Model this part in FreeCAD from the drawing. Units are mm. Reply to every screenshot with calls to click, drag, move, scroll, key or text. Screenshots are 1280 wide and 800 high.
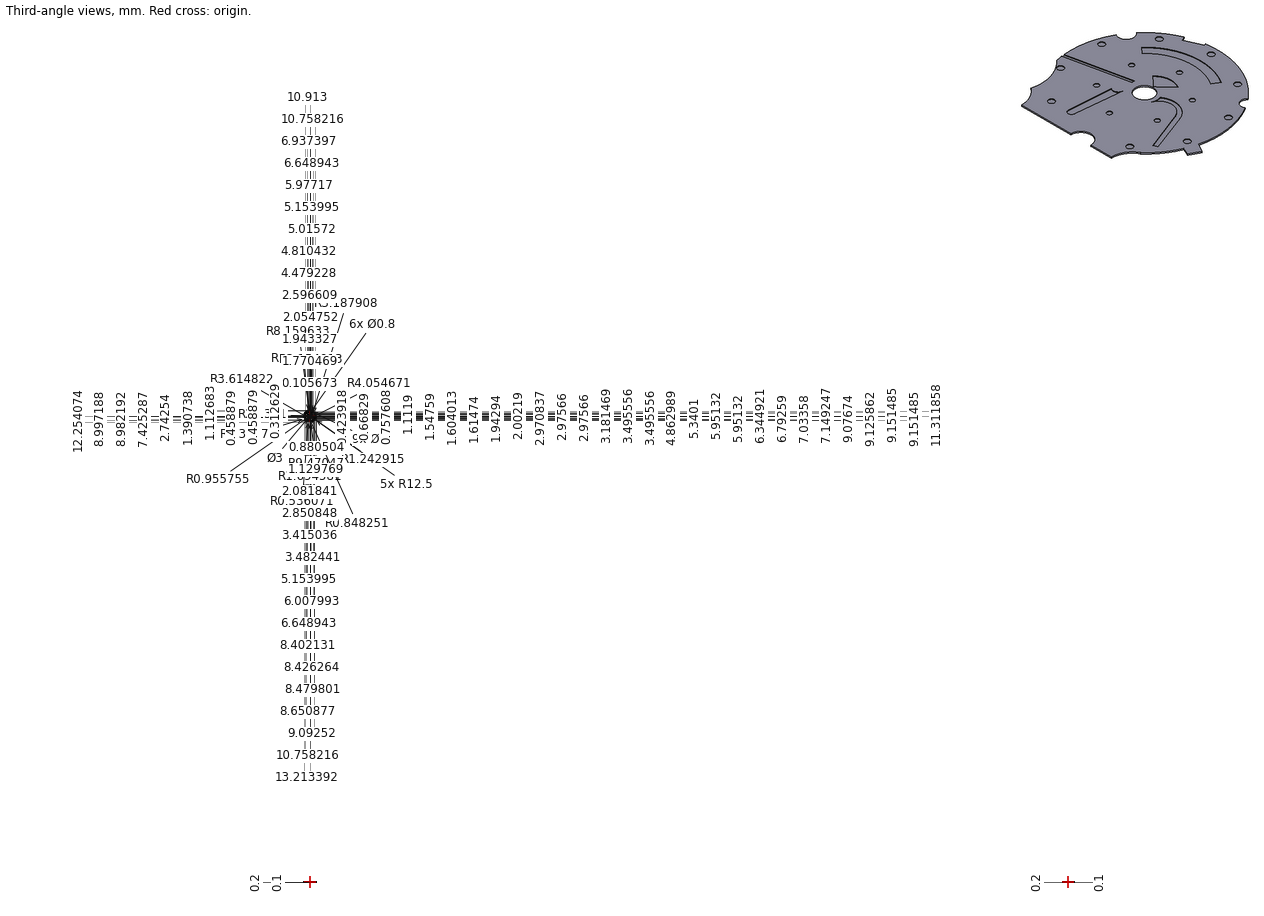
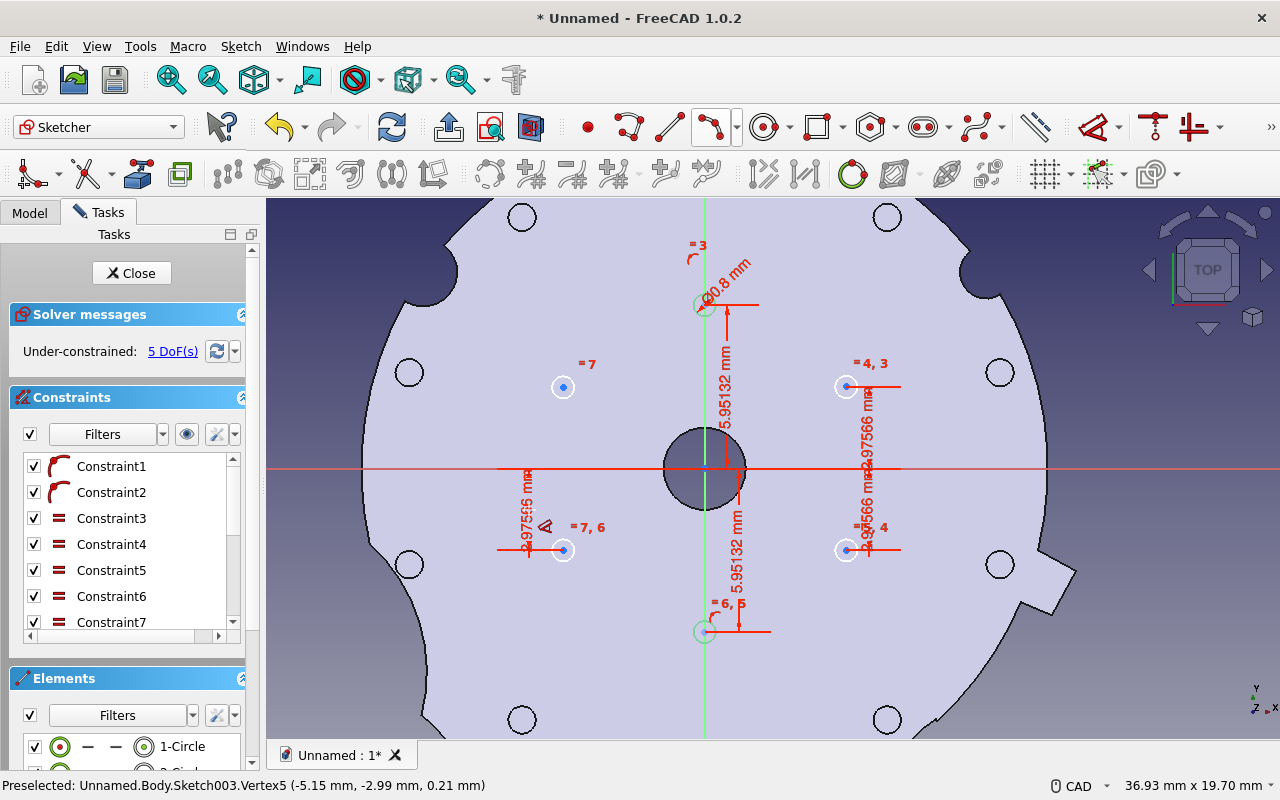
click(563, 387)
click(529, 428)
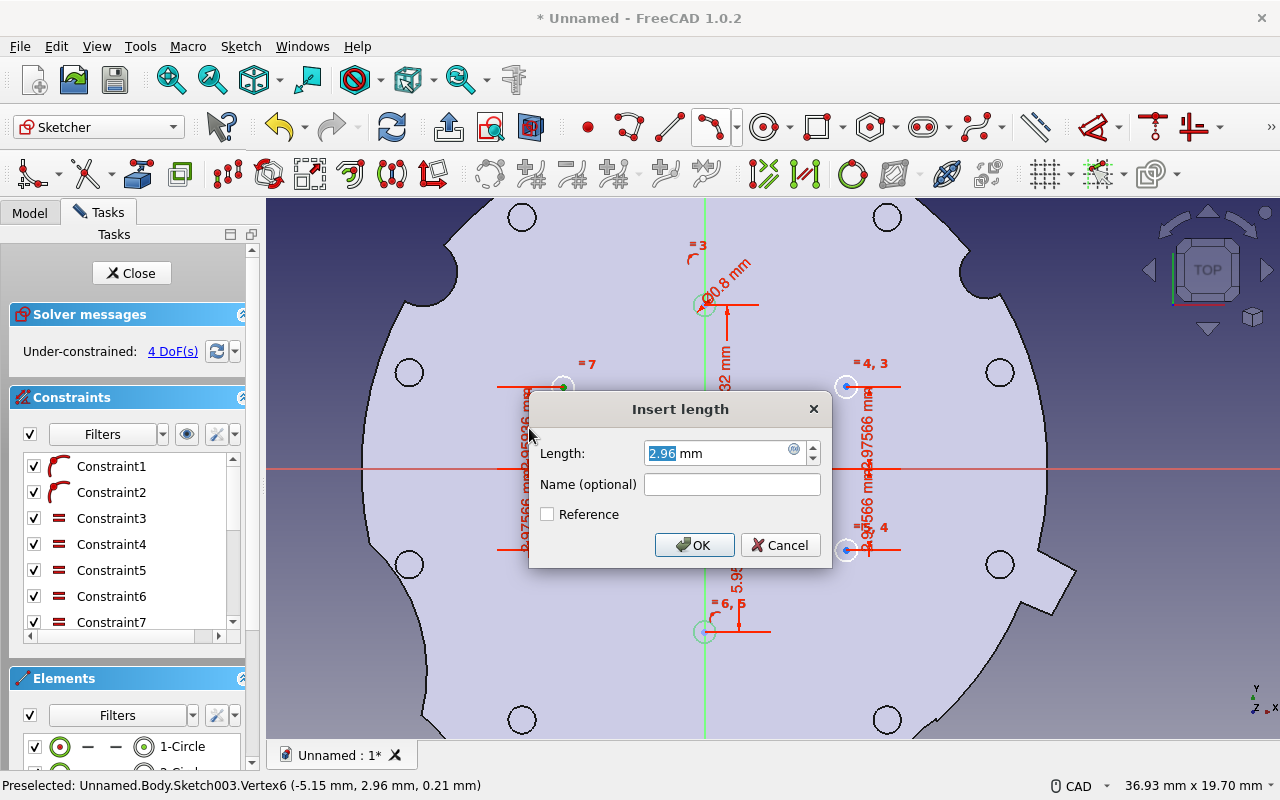
text(2.97566)
key(Return)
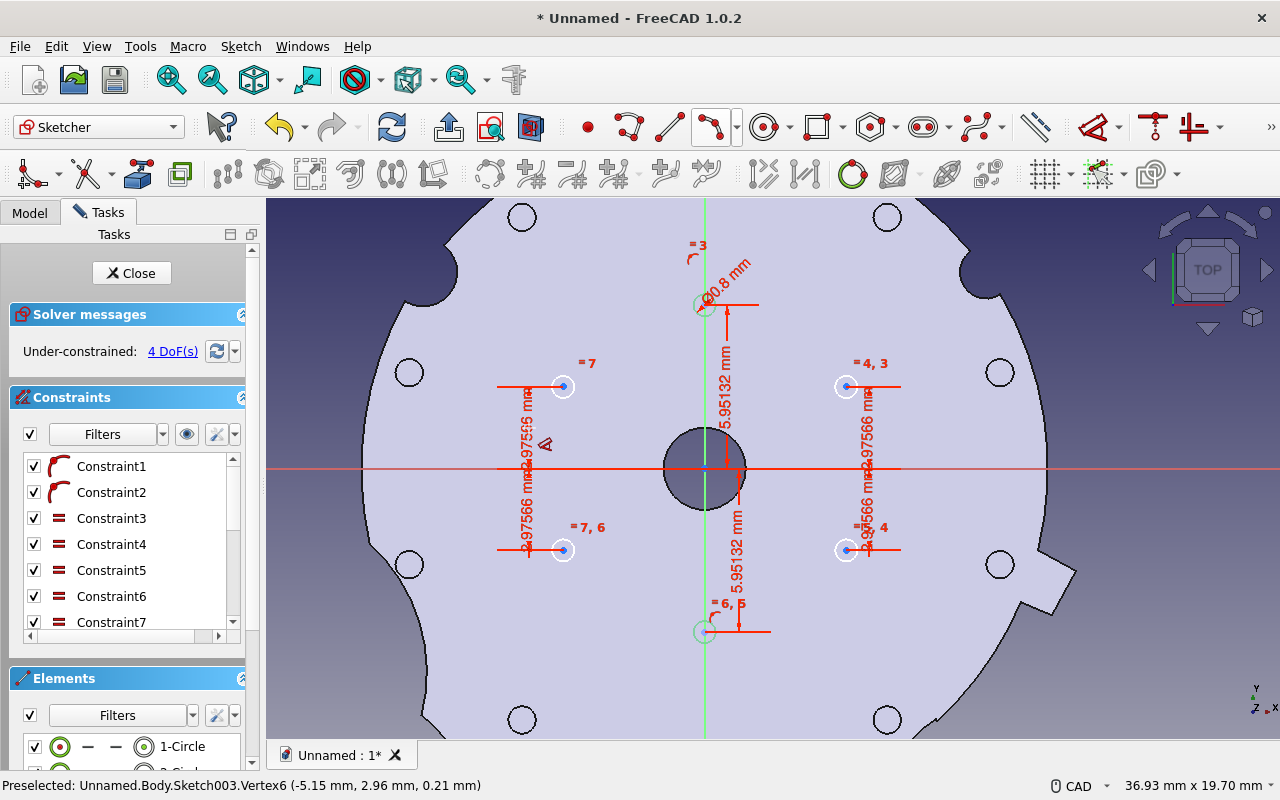
click(846, 387)
click(775, 353)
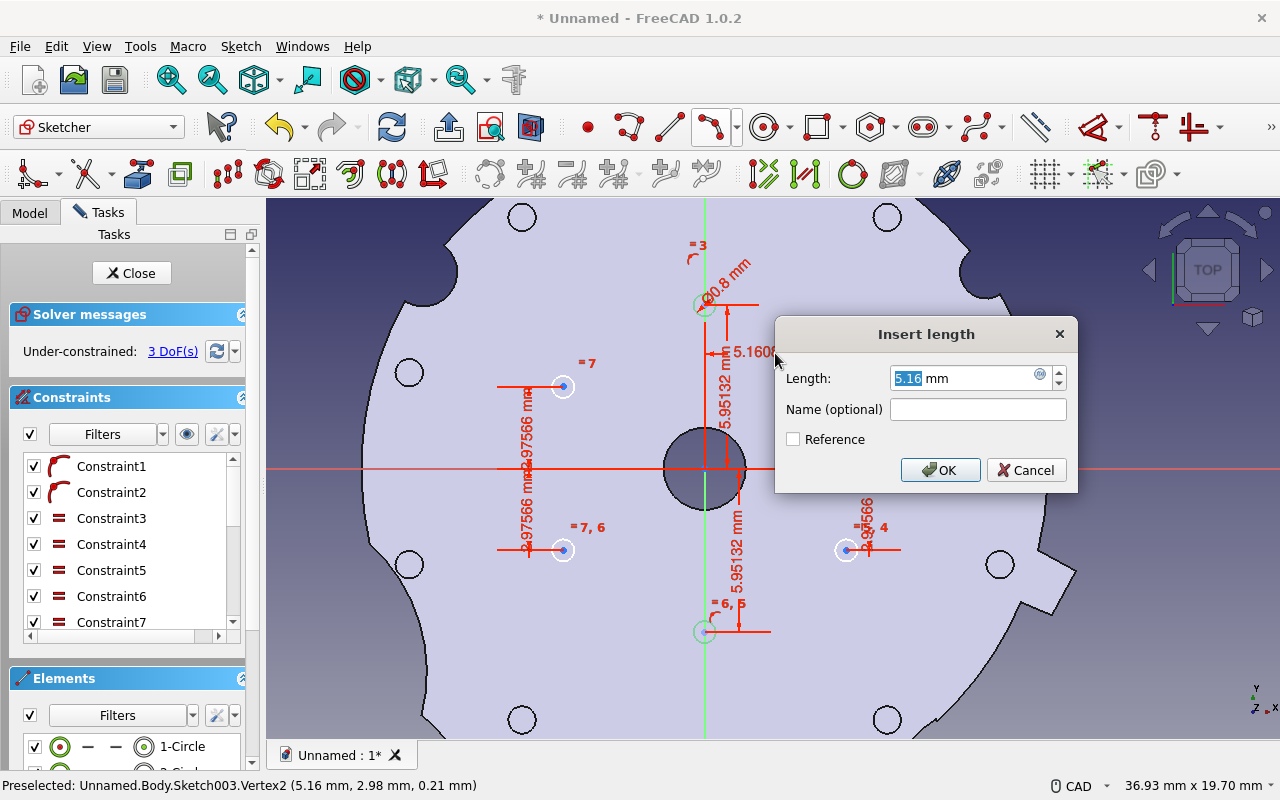
text(5.153995)
key(Return)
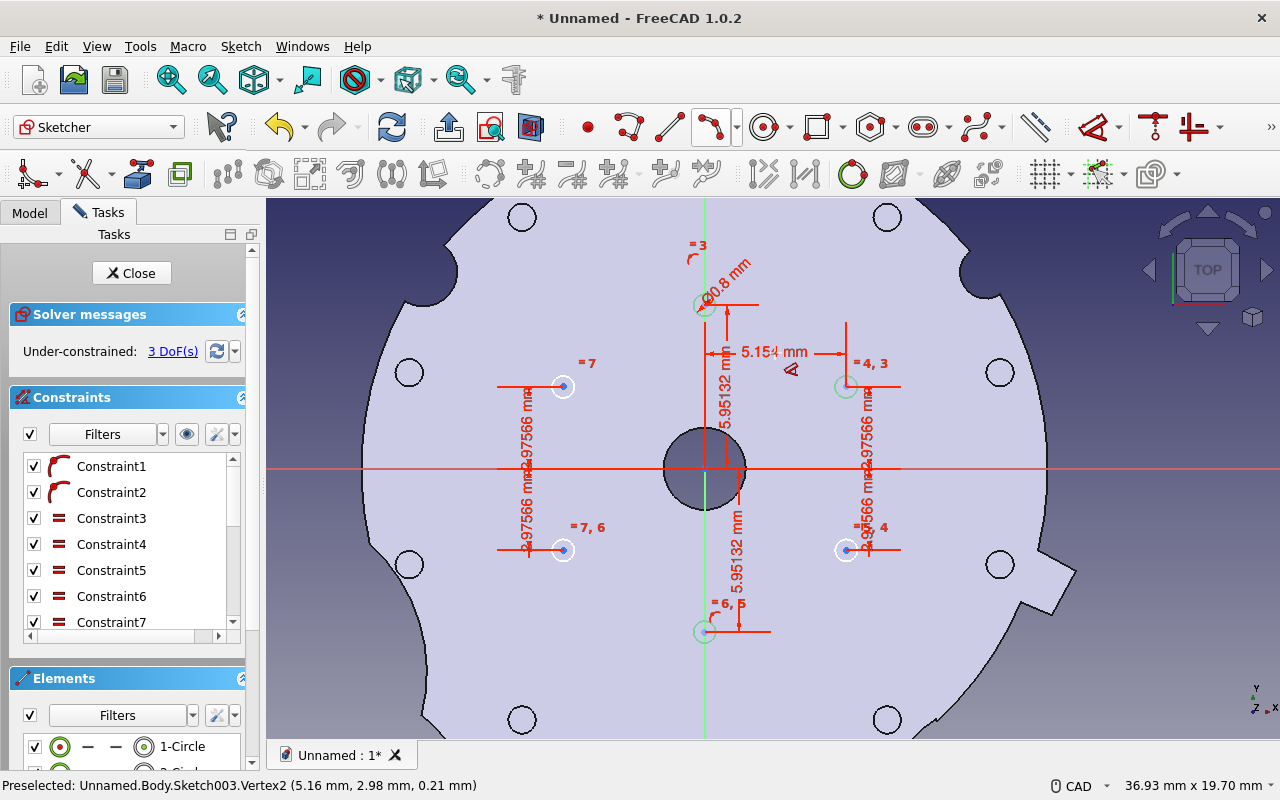
click(846, 550)
click(775, 584)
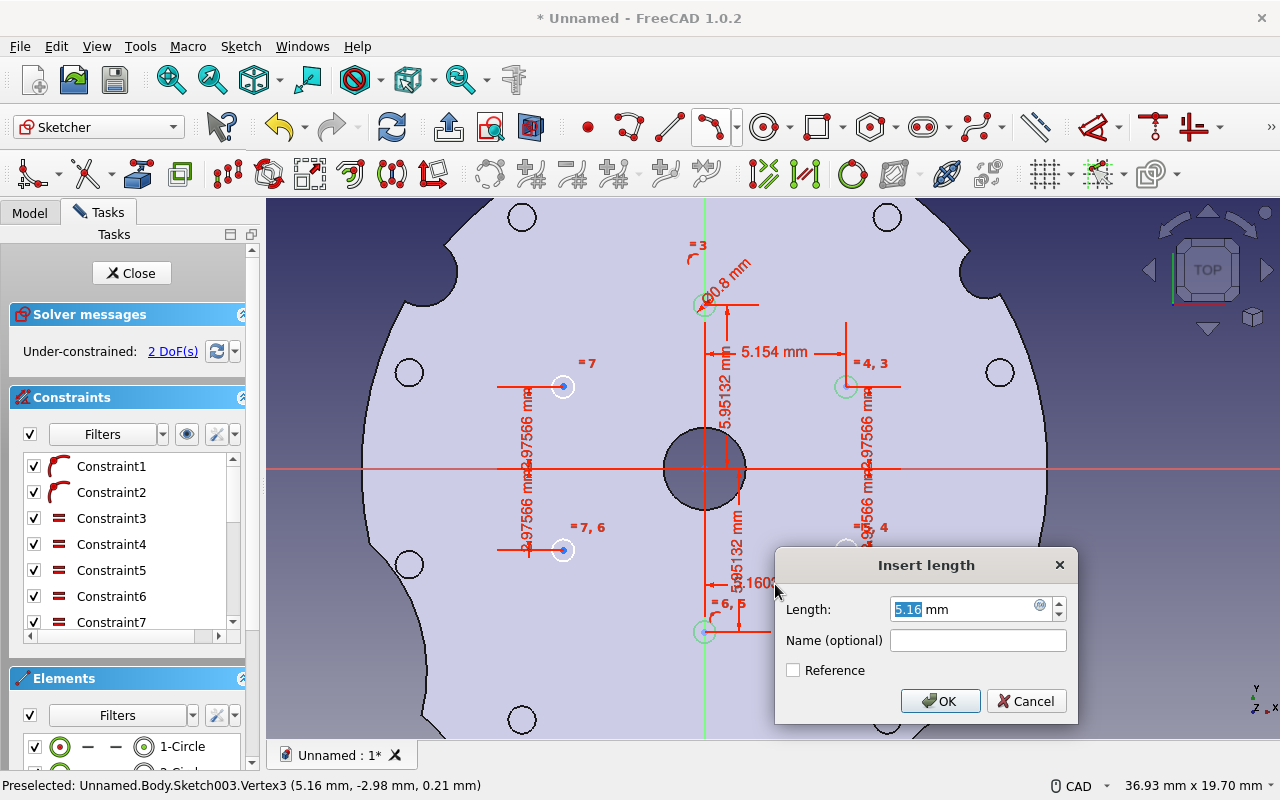
text(5.153995)
key(Return)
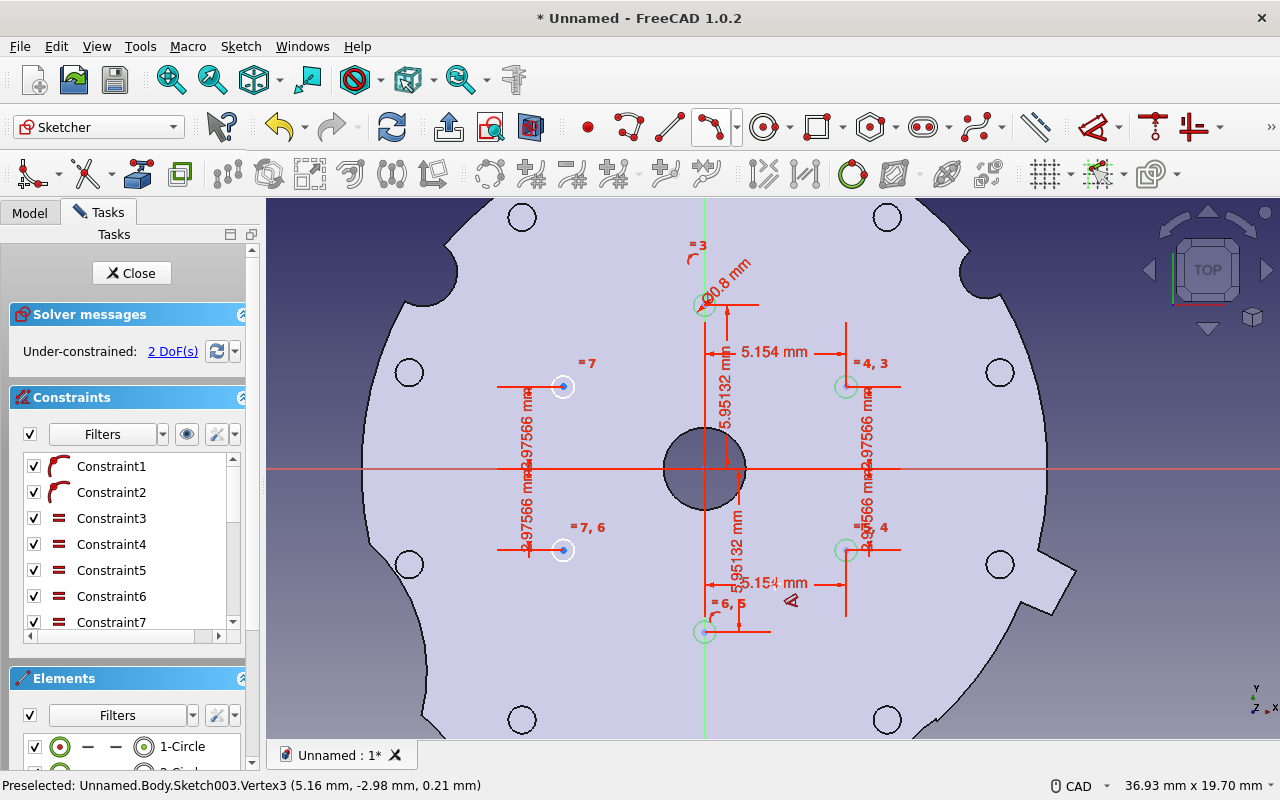
click(563, 550)
click(634, 584)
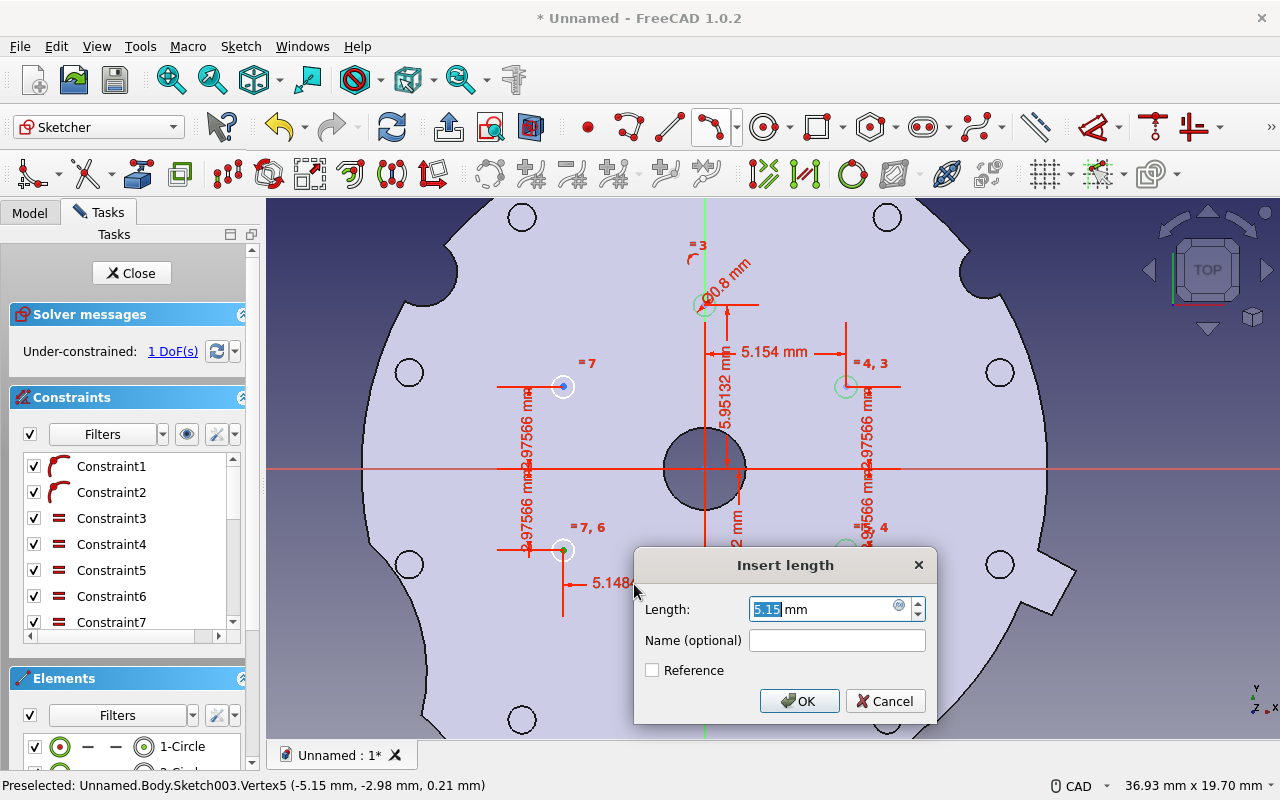
text(5.153995)
key(Return)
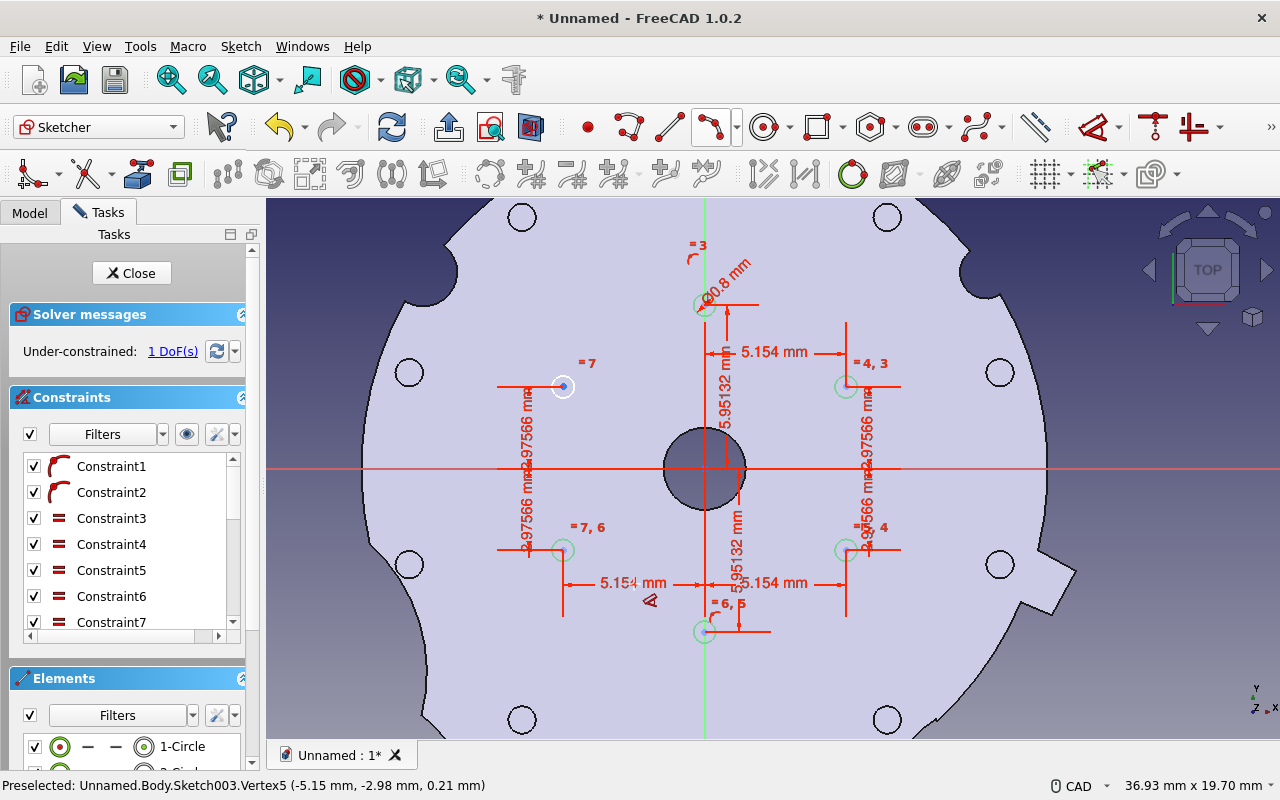
click(563, 387)
click(634, 353)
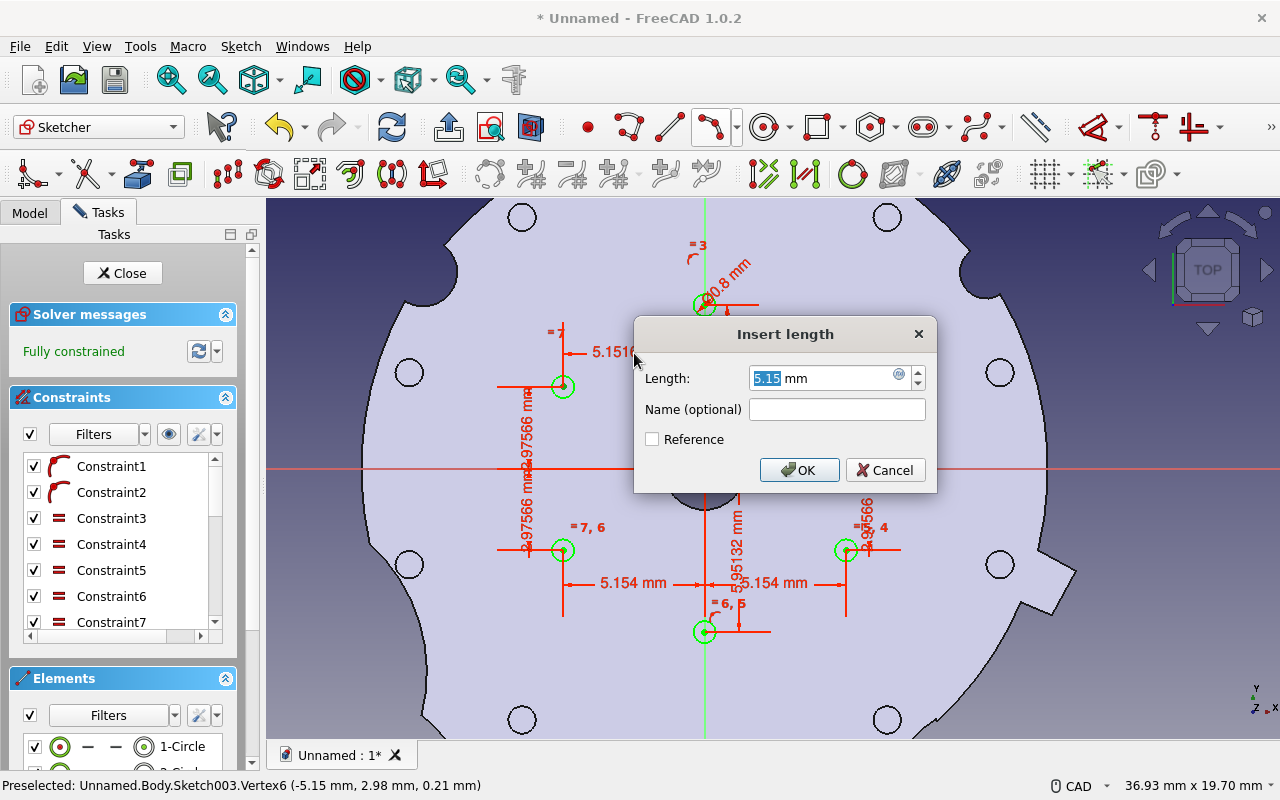
text(5.153995)
key(Return)
key(Escape)